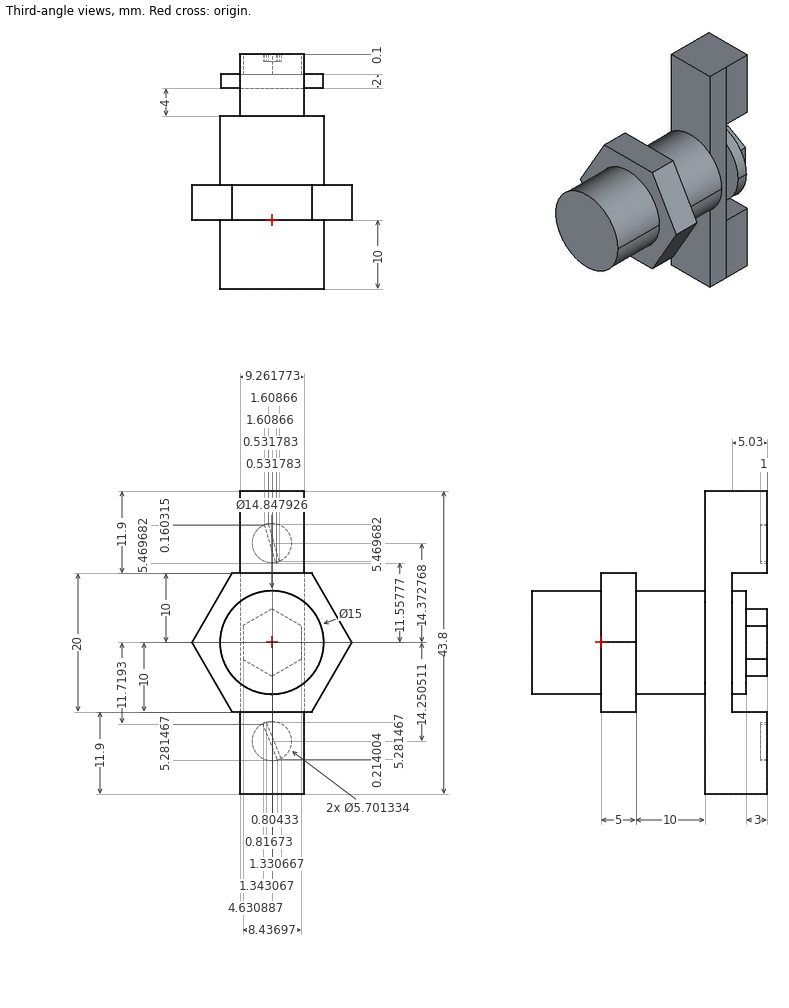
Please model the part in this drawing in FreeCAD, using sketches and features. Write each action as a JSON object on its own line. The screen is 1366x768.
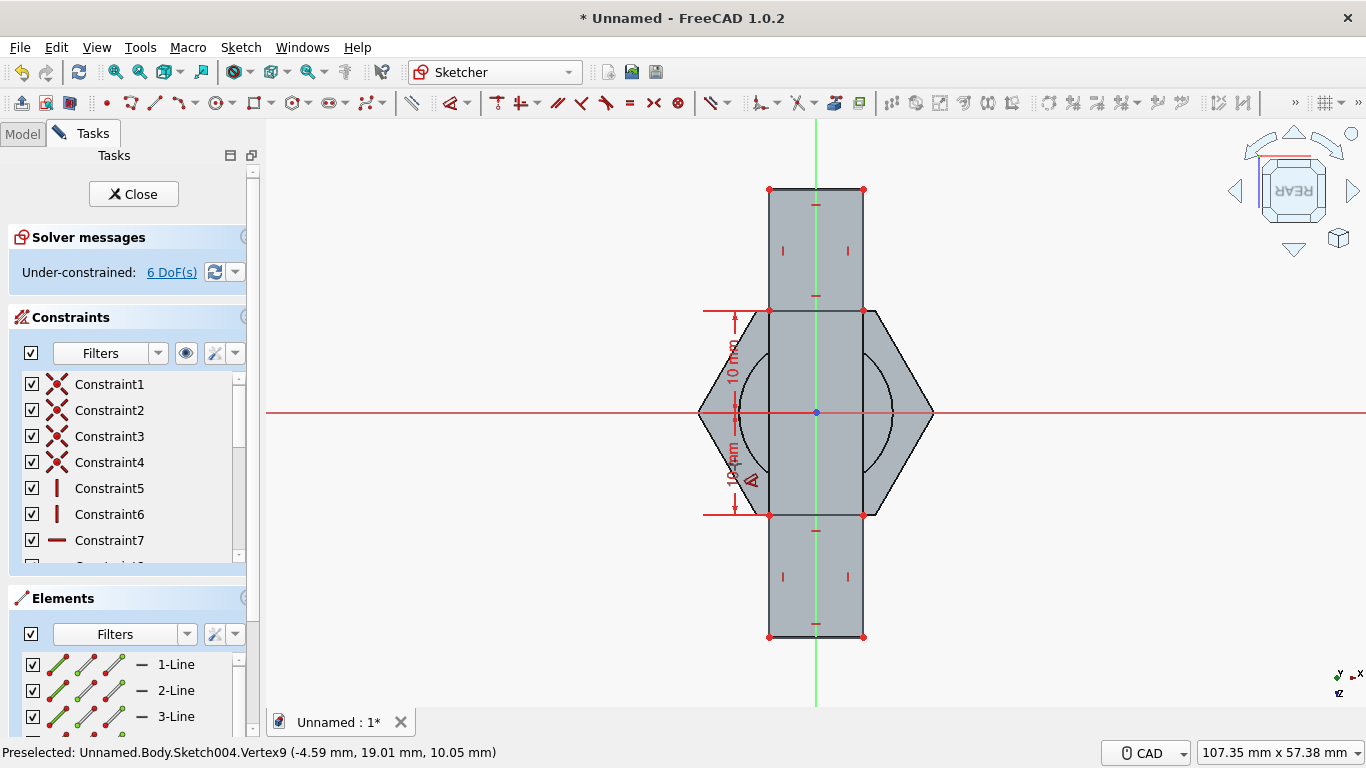
{"action": "left_click", "coordinate": [769, 226]}
{"action": "left_click", "coordinate": [735, 250]}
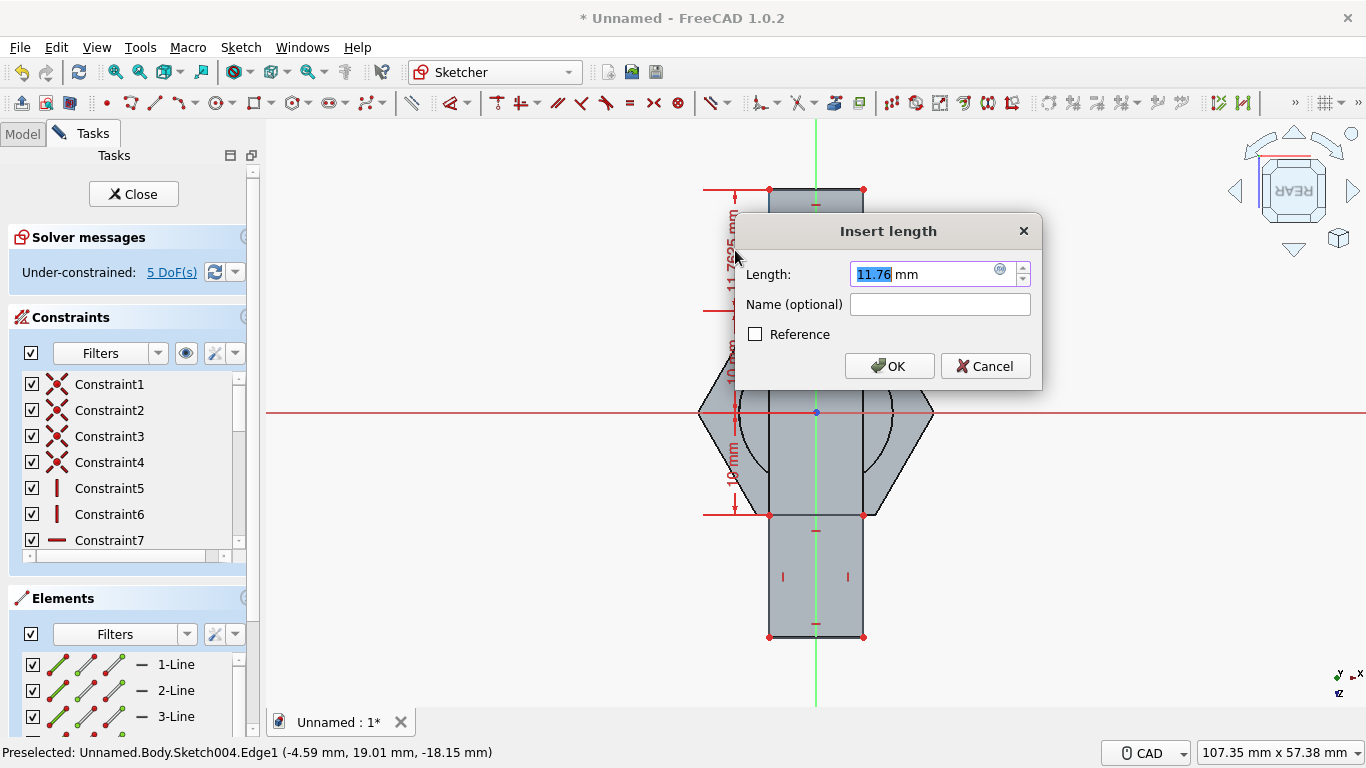
{"action": "type", "text": "11.9"}
{"action": "key", "text": "Return"}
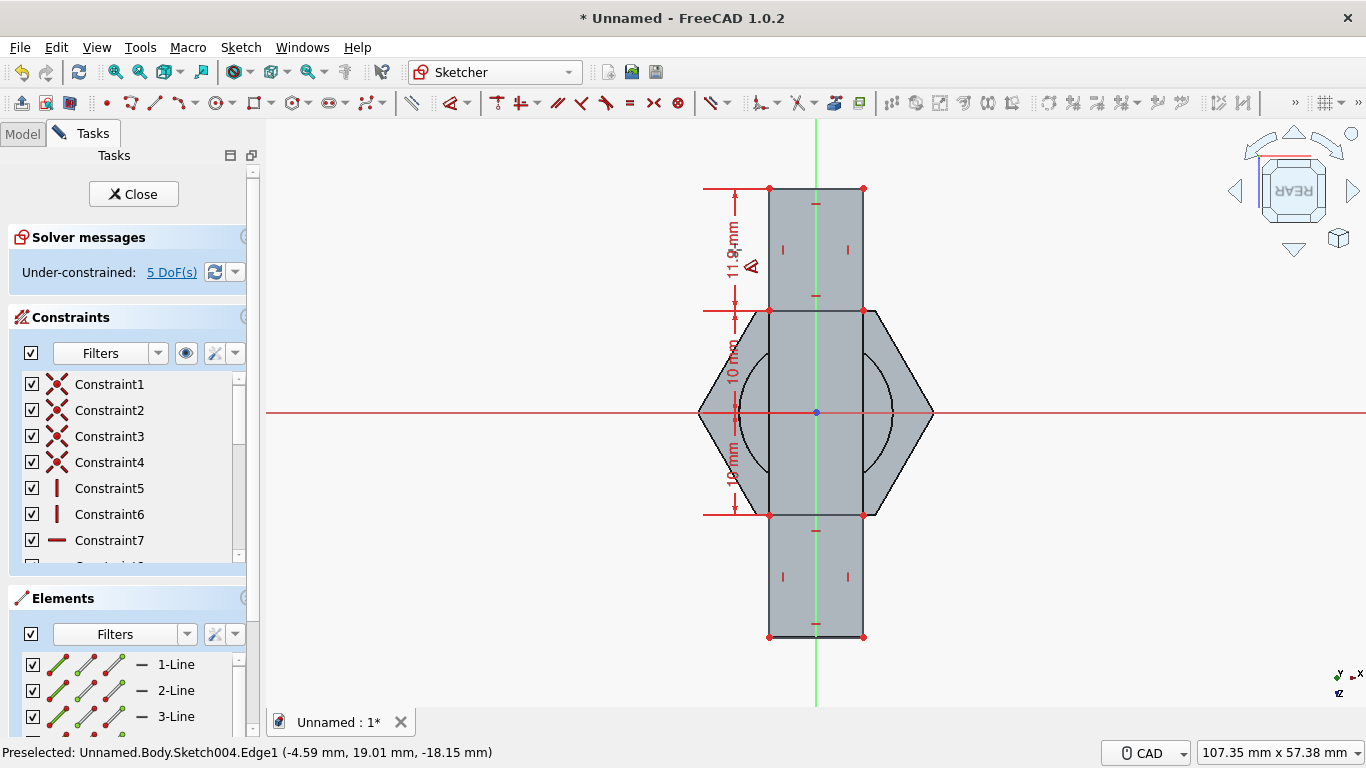
{"action": "left_click", "coordinate": [769, 552]}
{"action": "left_click", "coordinate": [735, 577]}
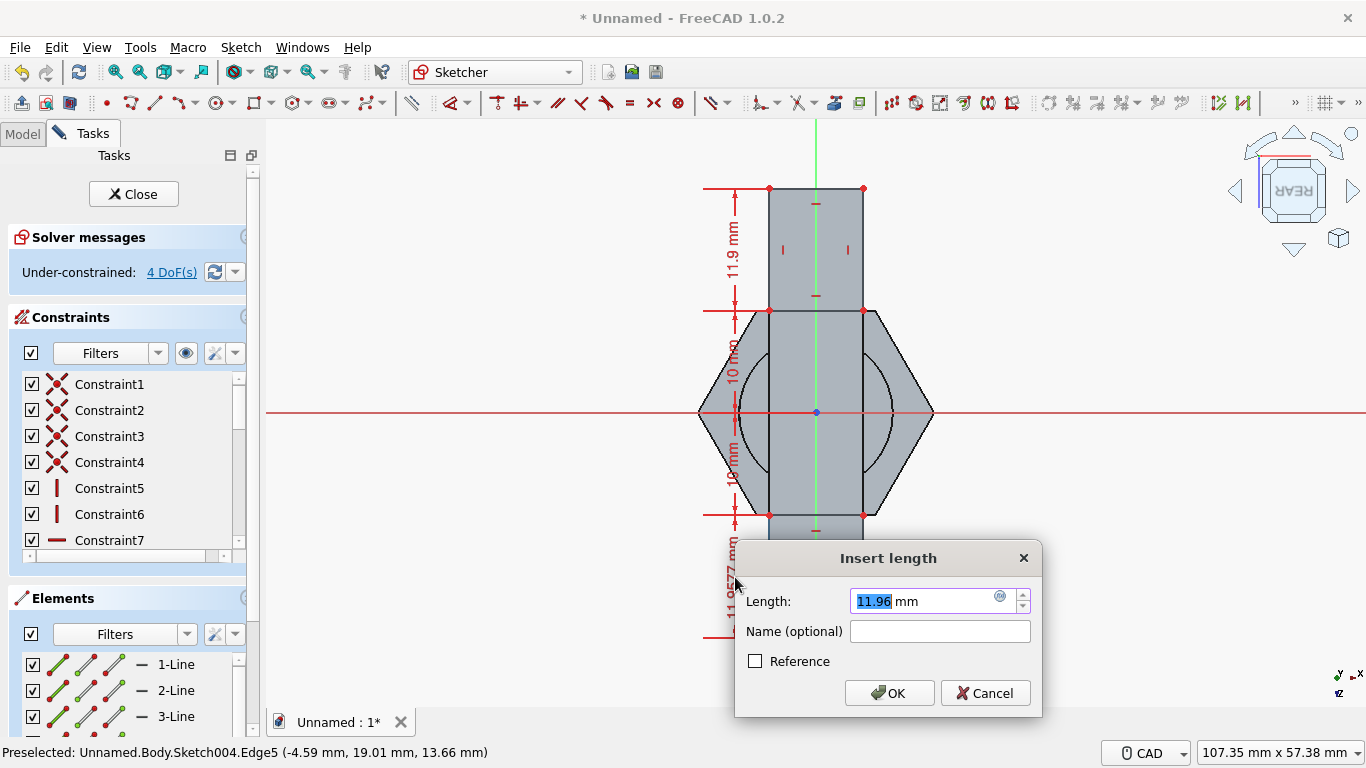
{"action": "type", "text": "11.9"}
{"action": "key", "text": "Return"}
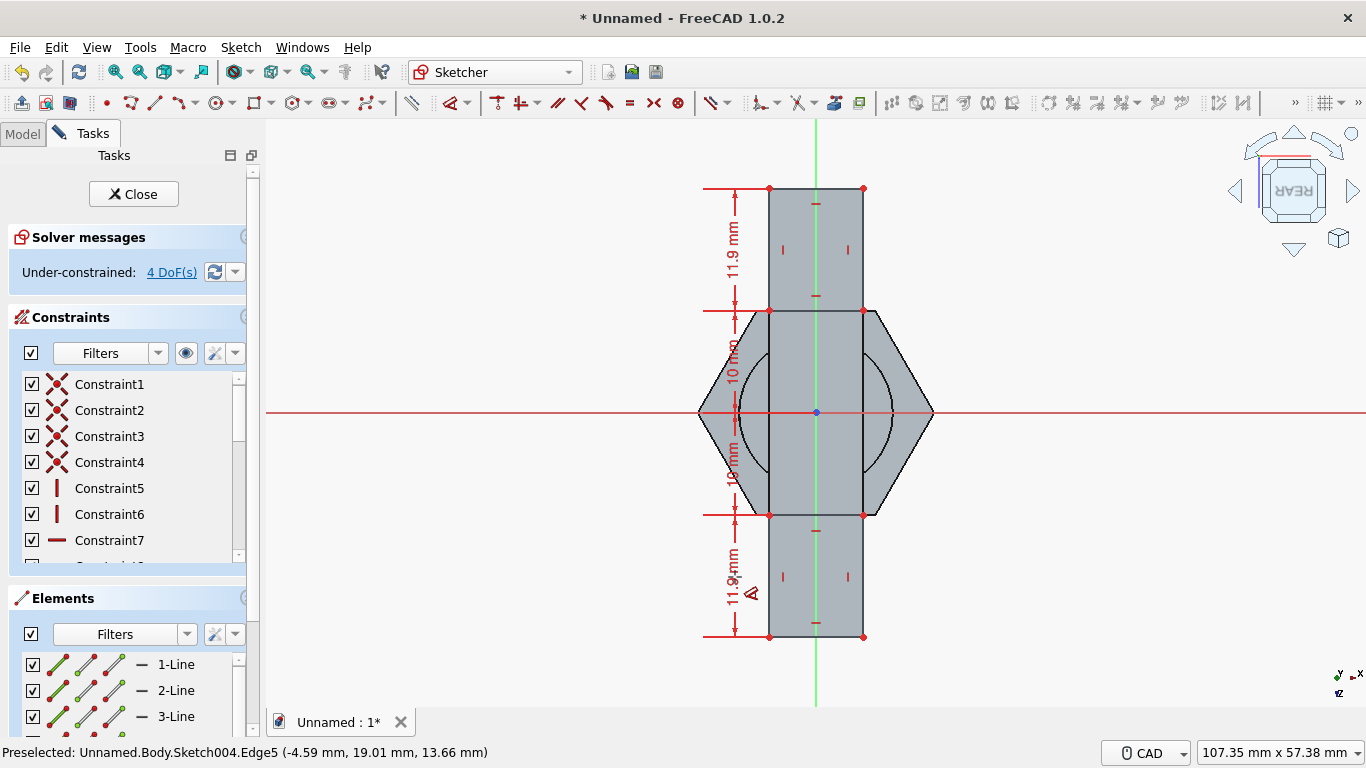
{"action": "left_click", "coordinate": [797, 311]}
{"action": "left_click", "coordinate": [794, 277]}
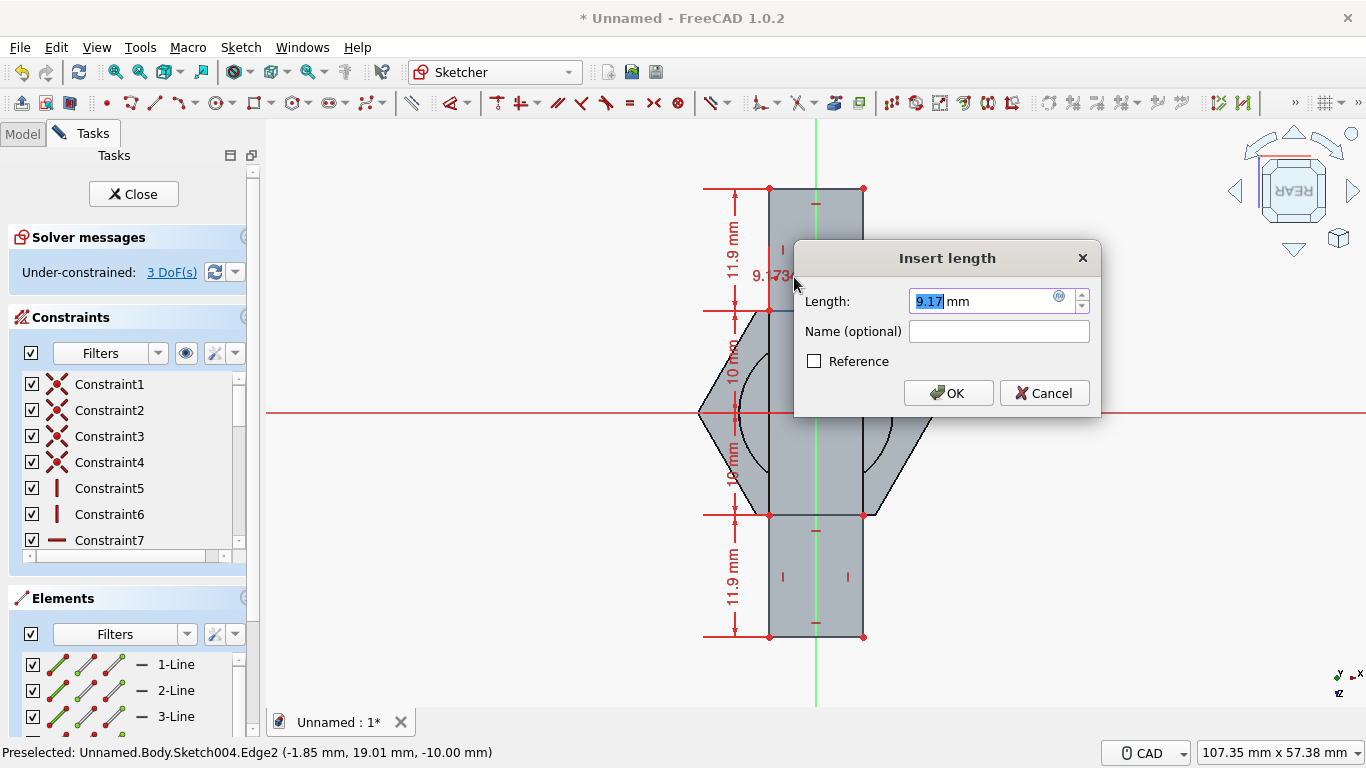
{"action": "type", "text": "9.261773"}
{"action": "key", "text": "Return"}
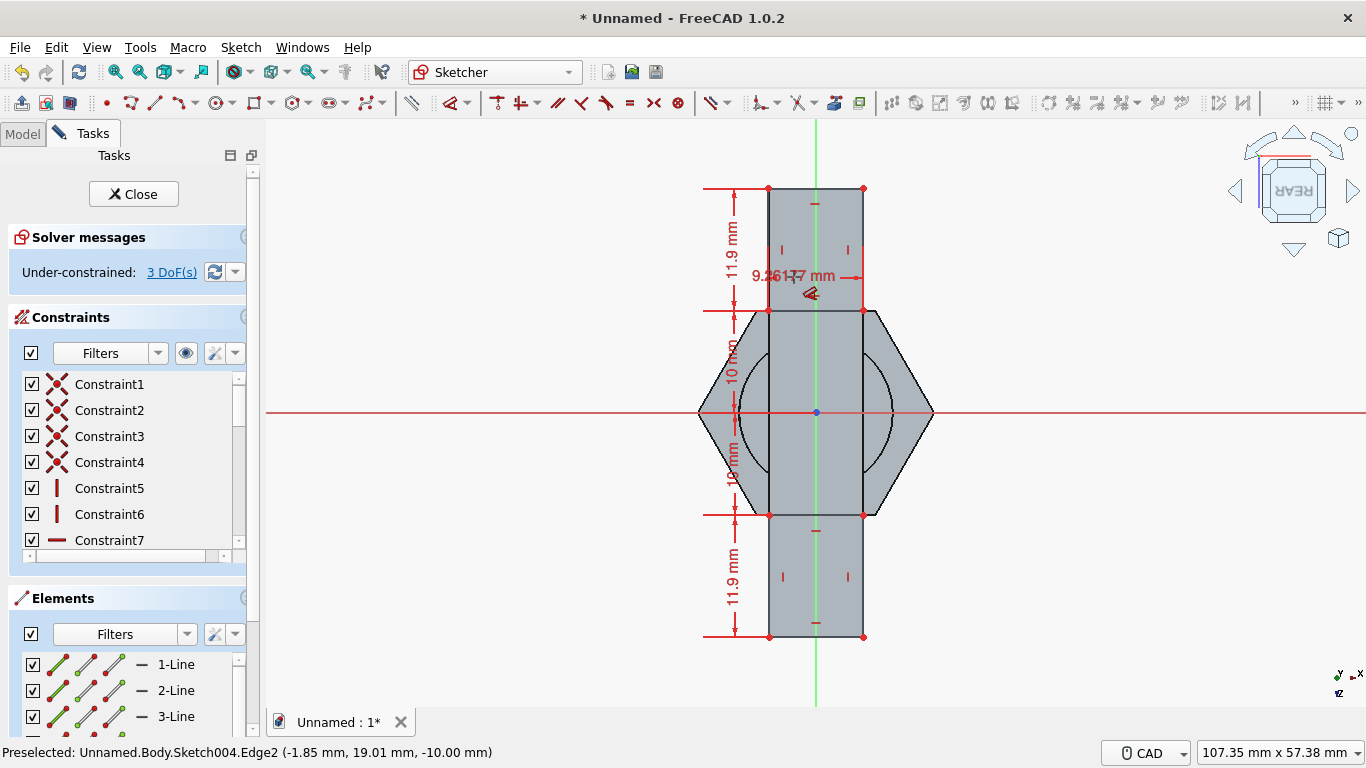
{"action": "left_click", "coordinate": [797, 637]}
{"action": "left_click", "coordinate": [794, 671]}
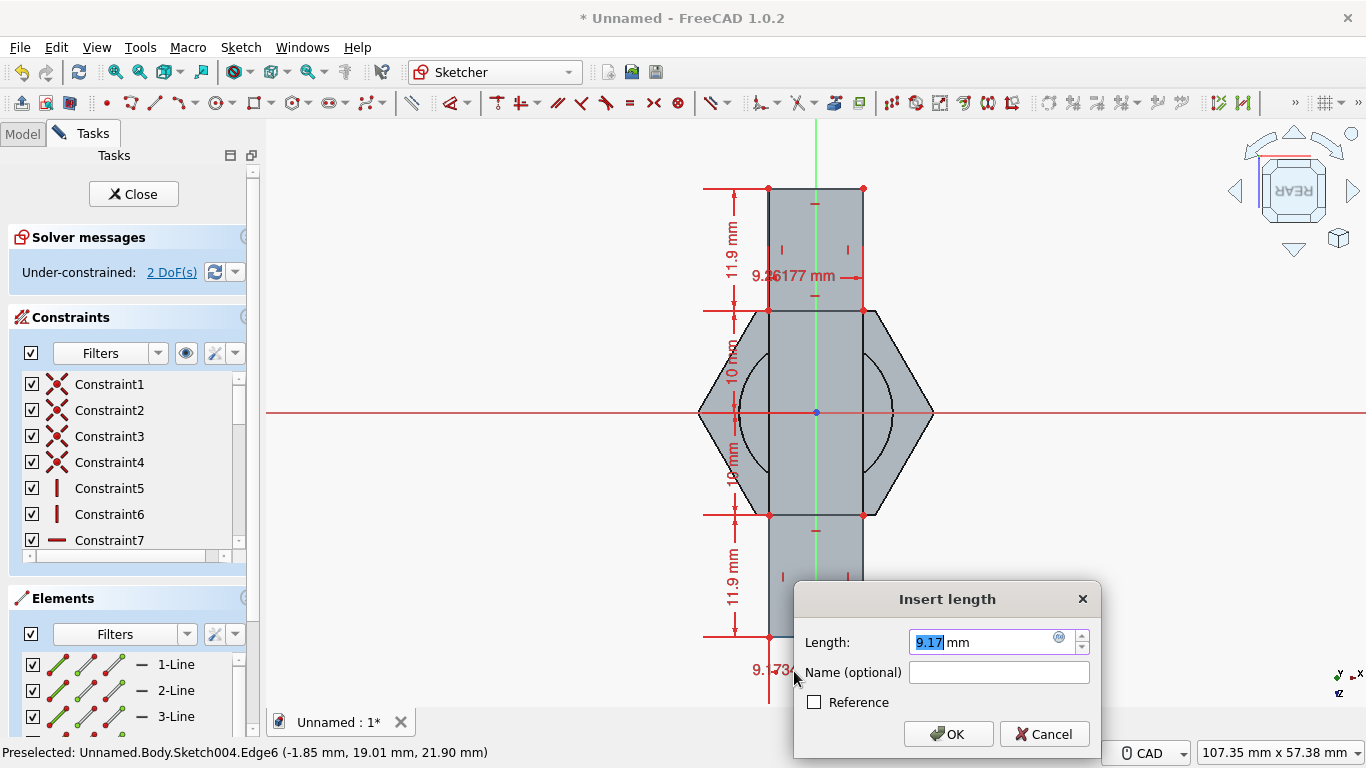
{"action": "type", "text": "9.261773"}
{"action": "key", "text": "Return"}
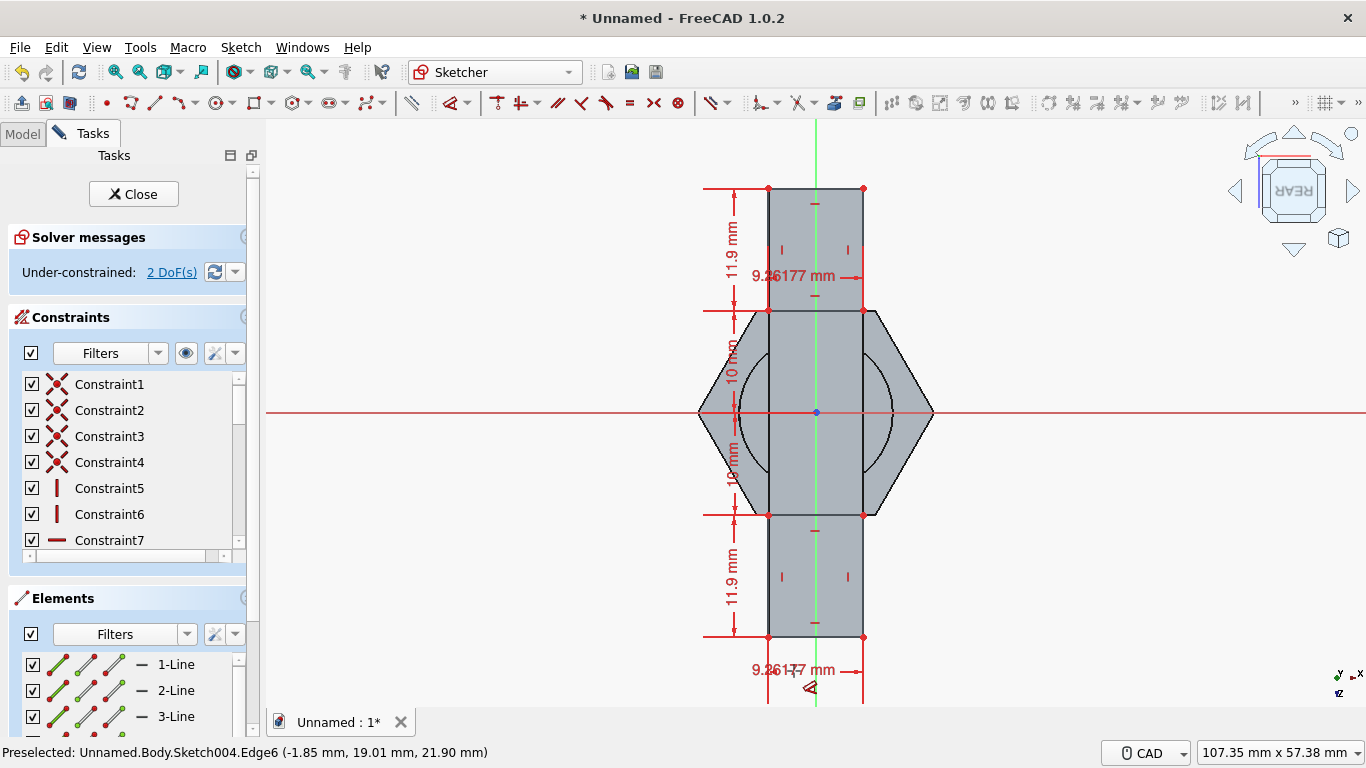
{"action": "left_click", "coordinate": [768, 189]}
{"action": "left_click", "coordinate": [792, 155]}